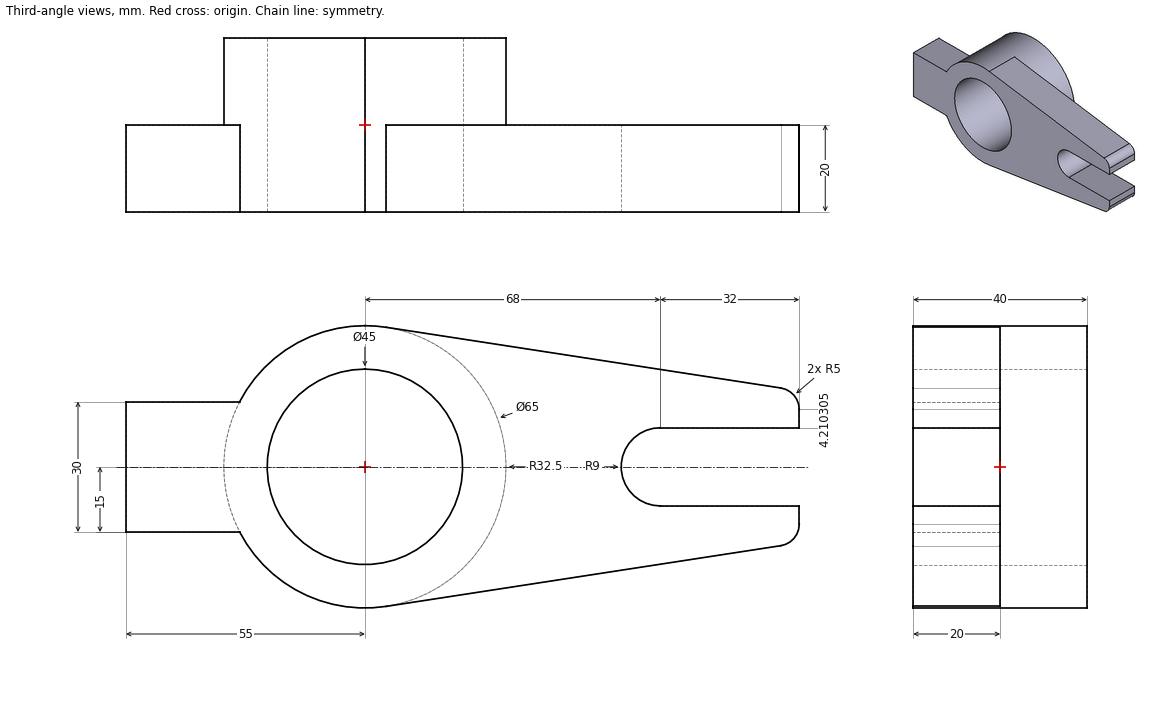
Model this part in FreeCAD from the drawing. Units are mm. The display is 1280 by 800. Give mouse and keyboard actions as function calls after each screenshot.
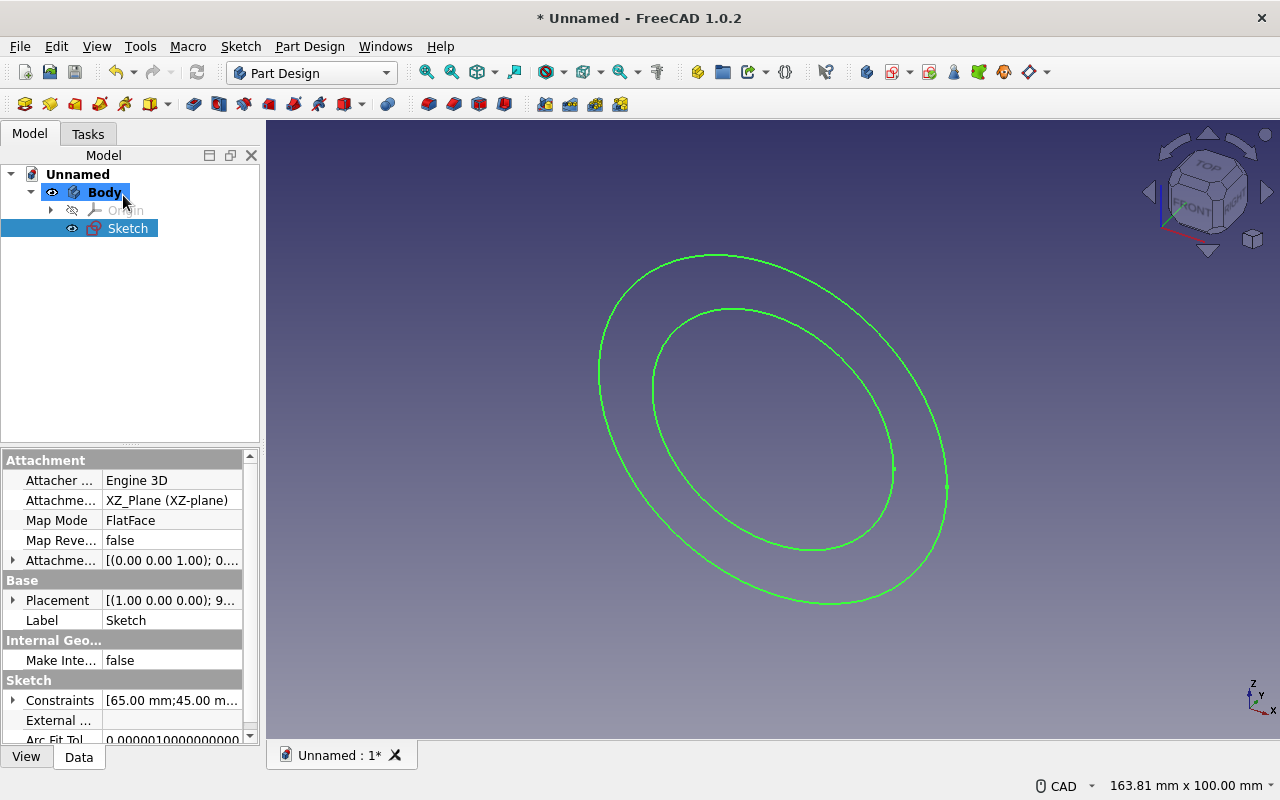
click(25, 104)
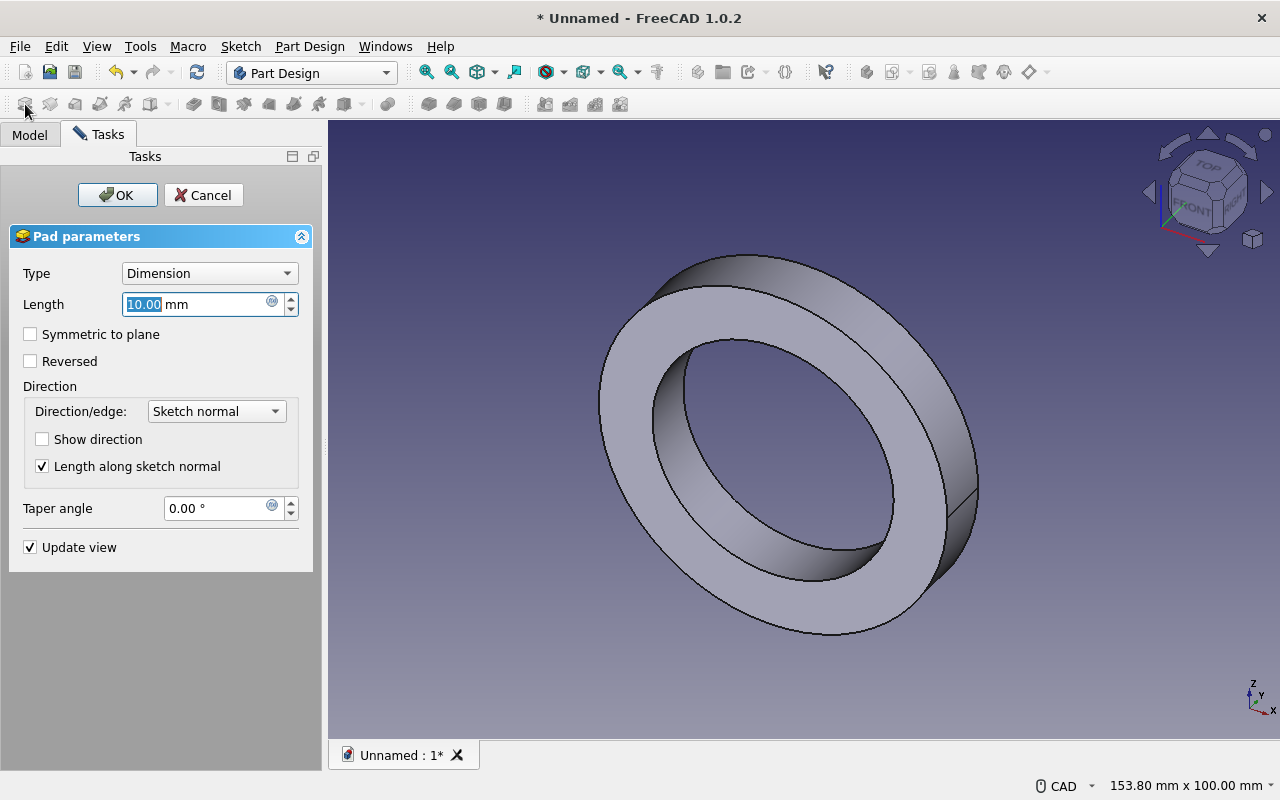
text(40)
key(Tab)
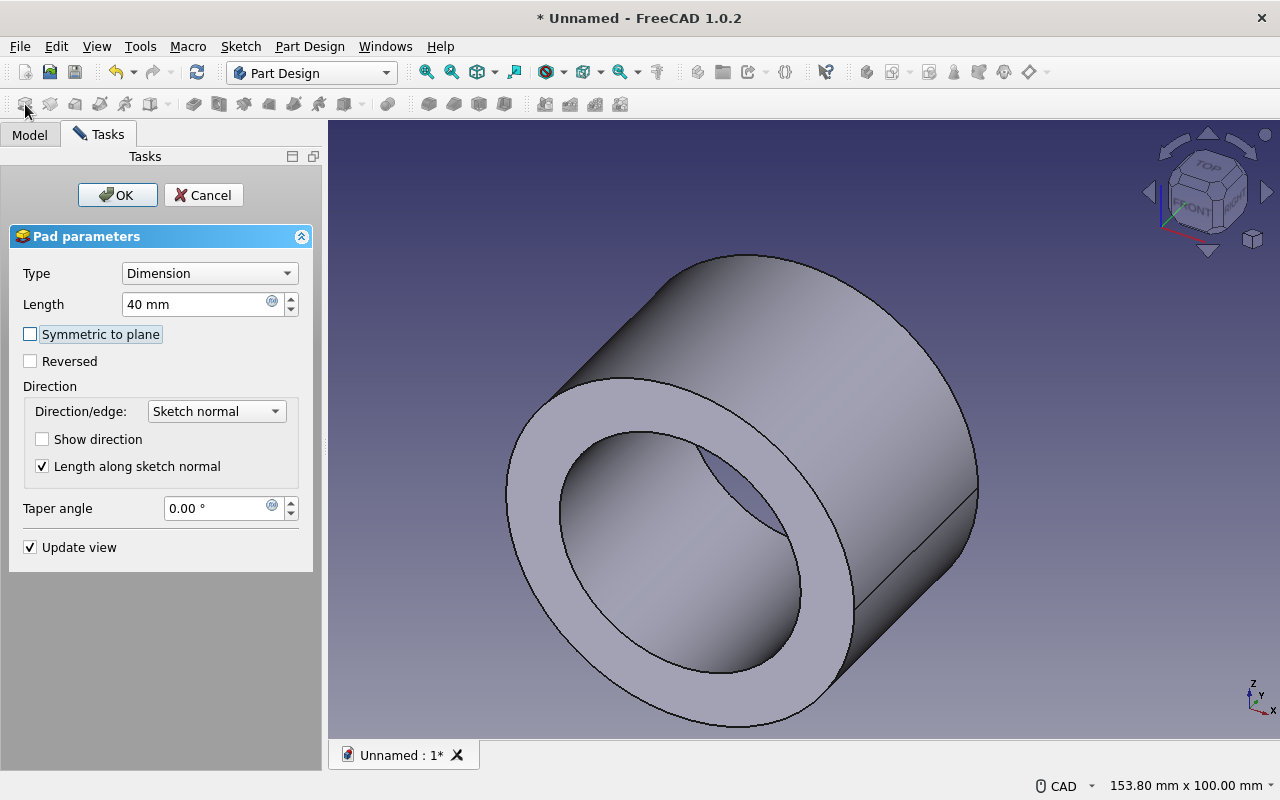
click(31, 334)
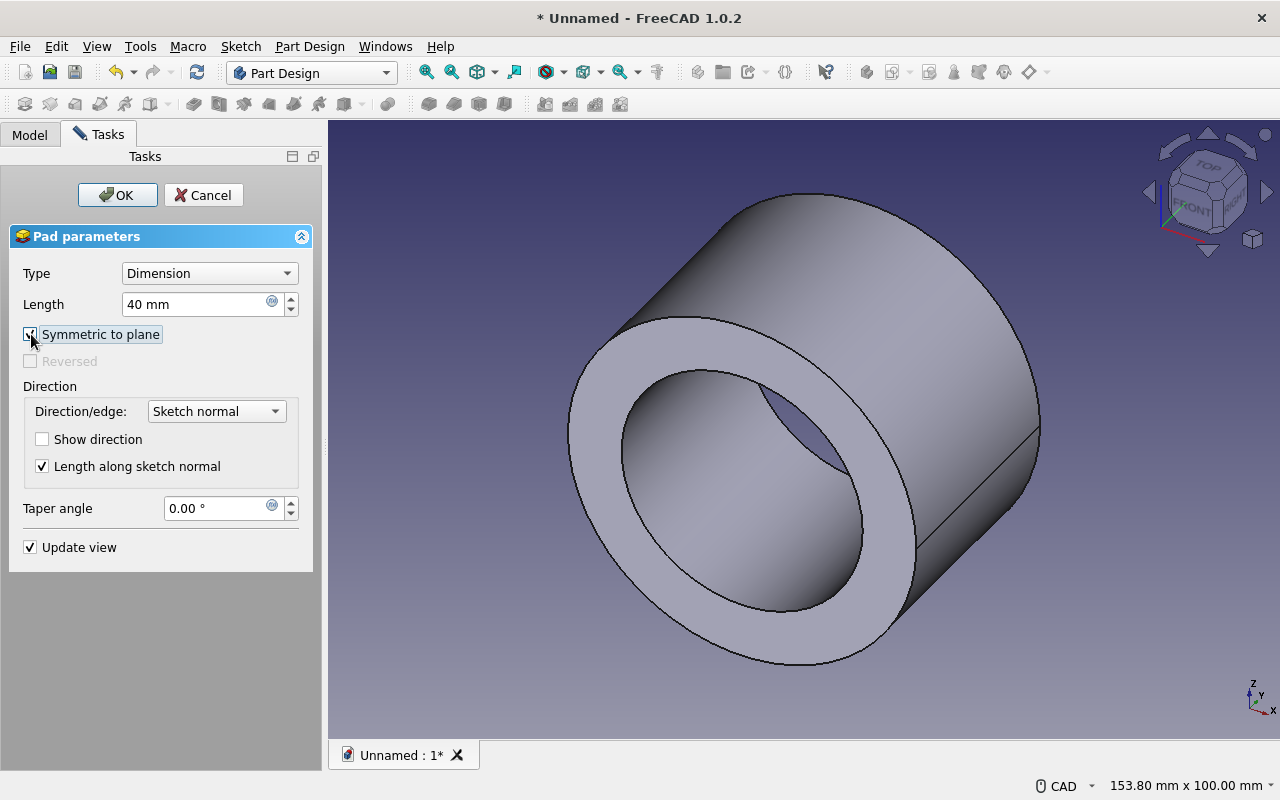
click(118, 195)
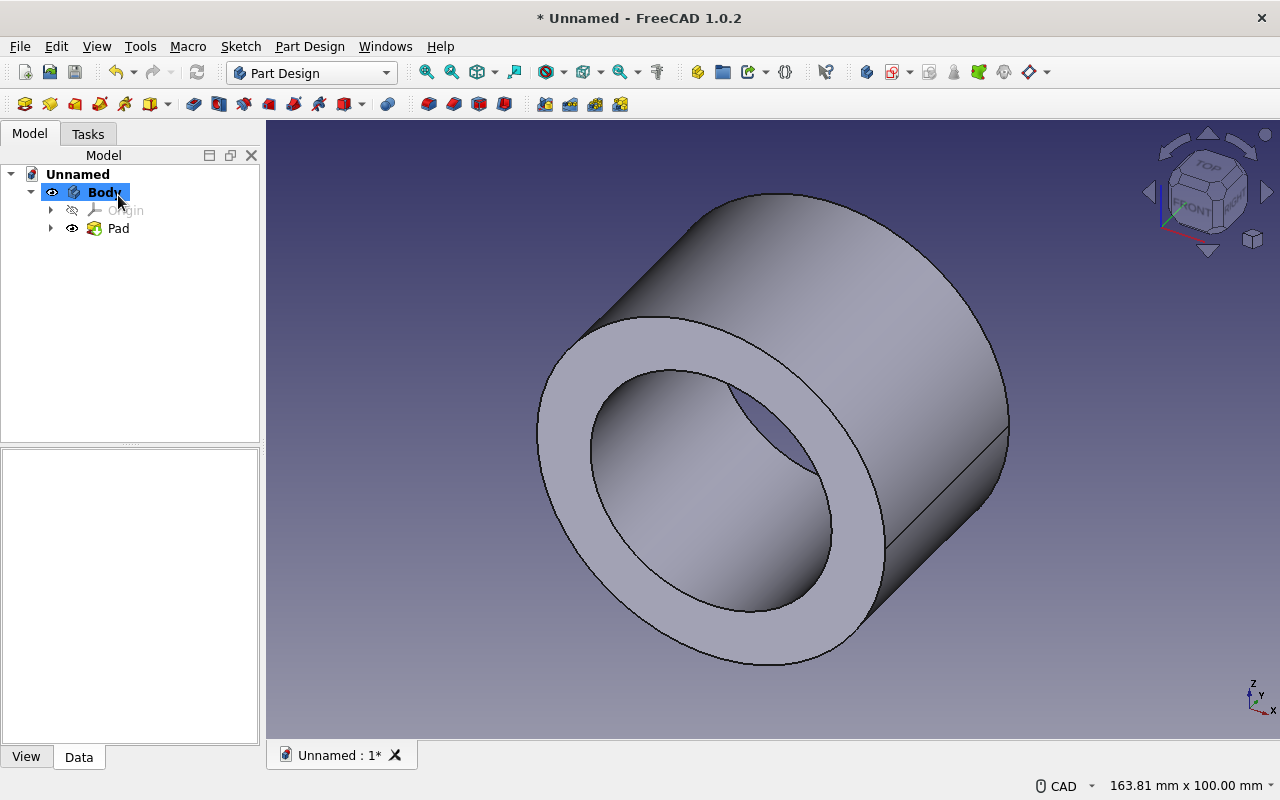
click(892, 72)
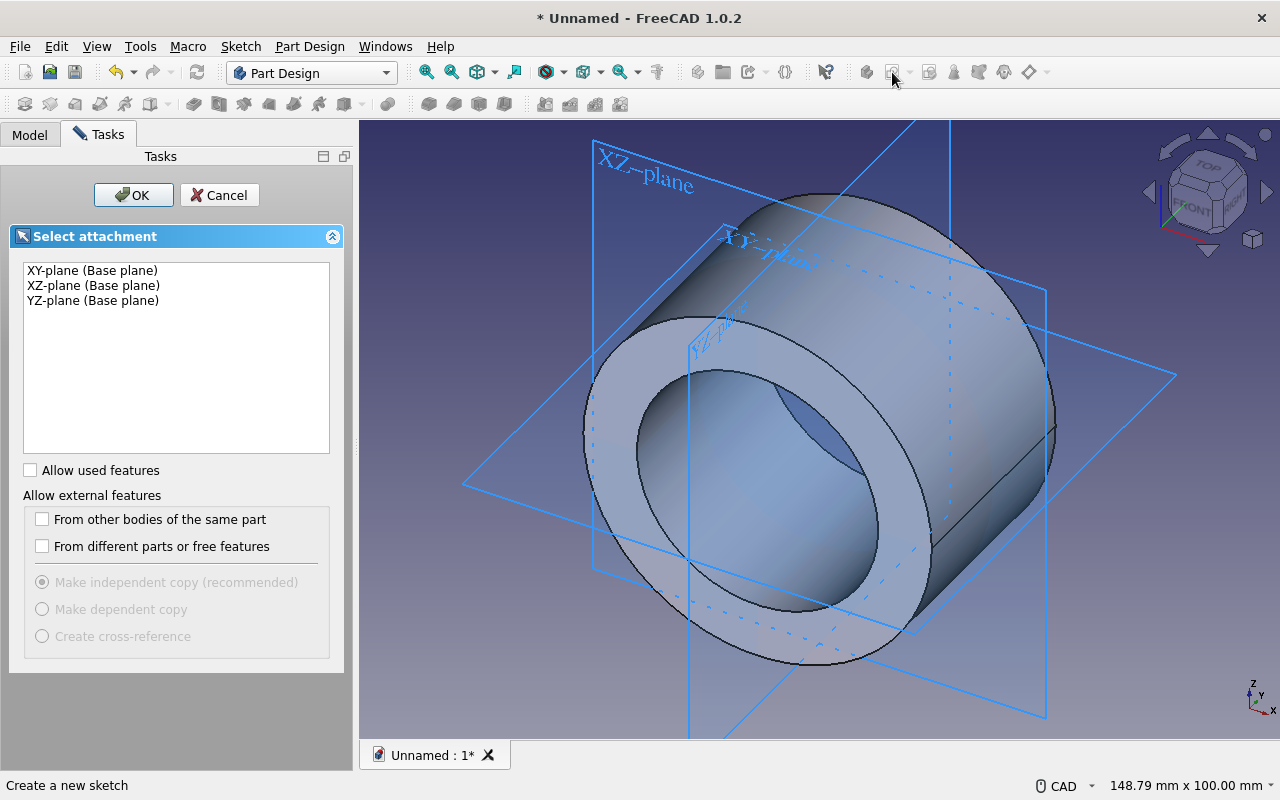
click(84, 286)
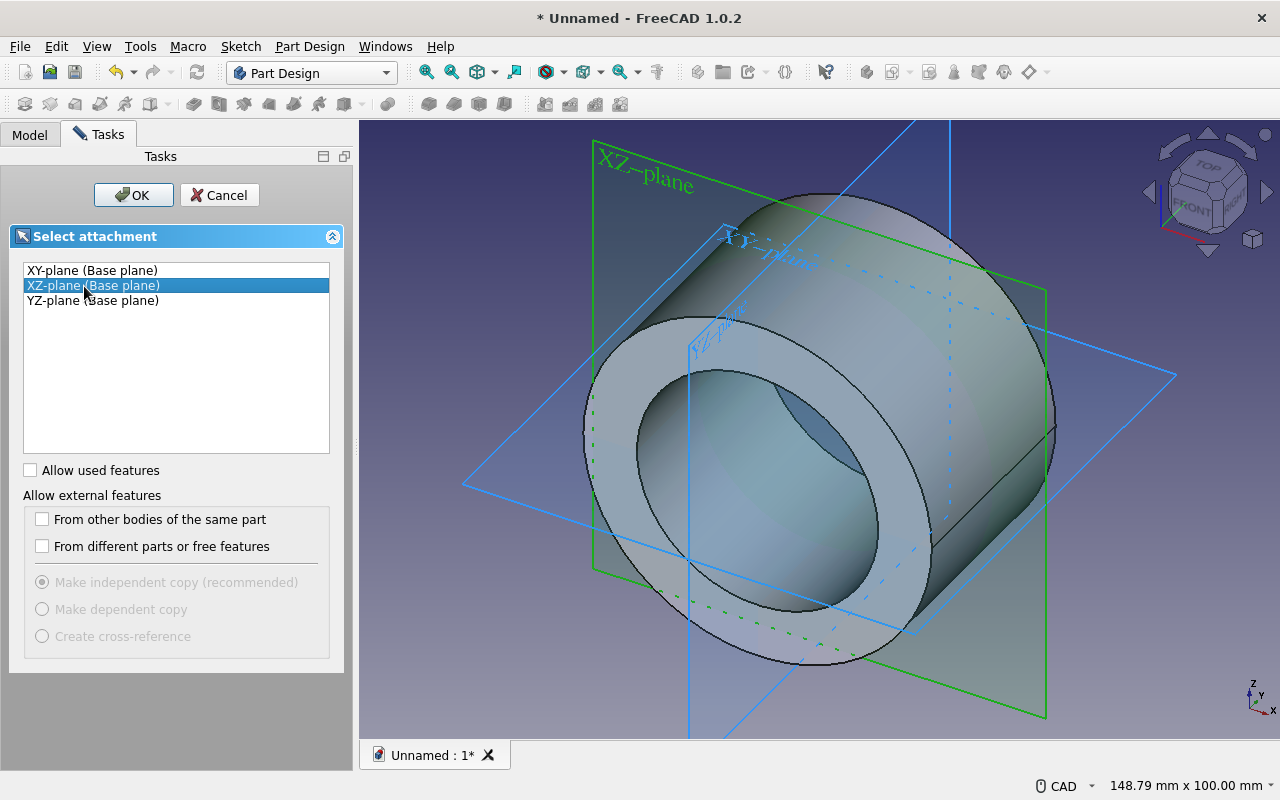
click(134, 195)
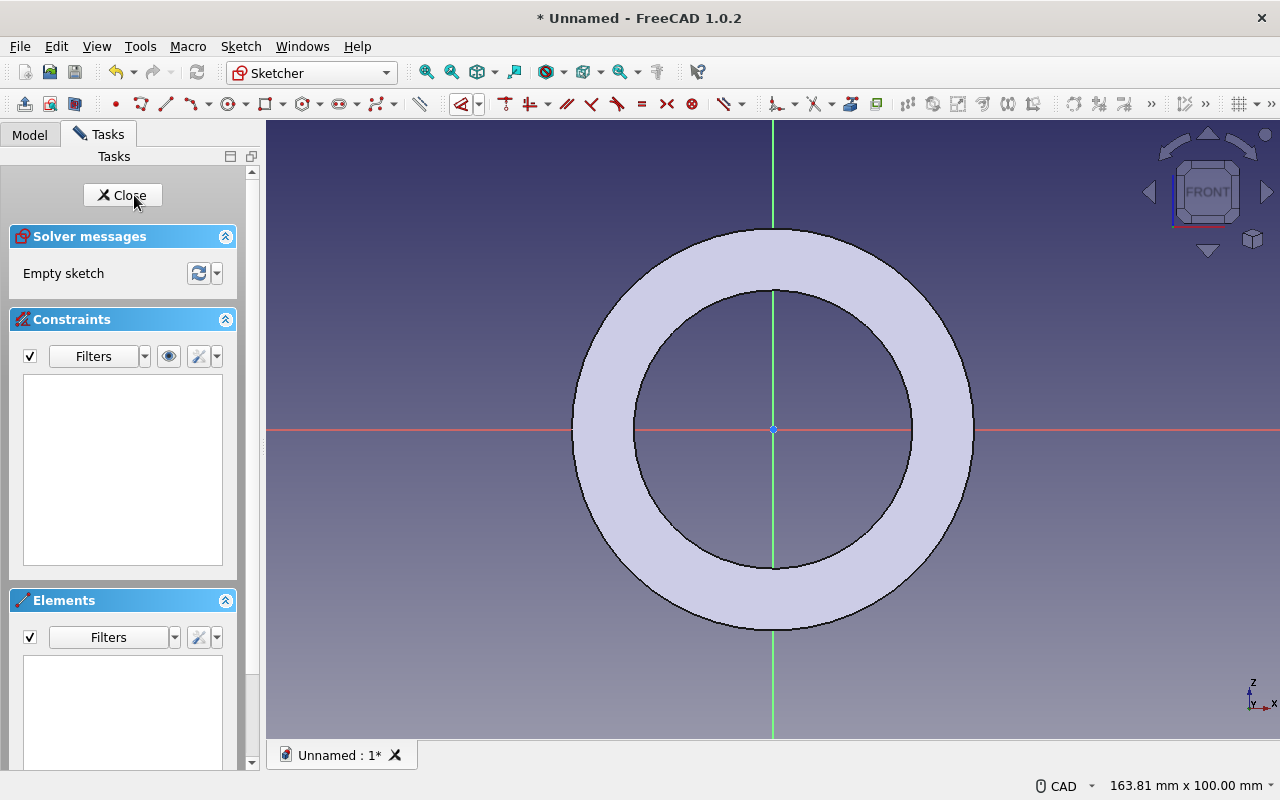
key(q)
key(s)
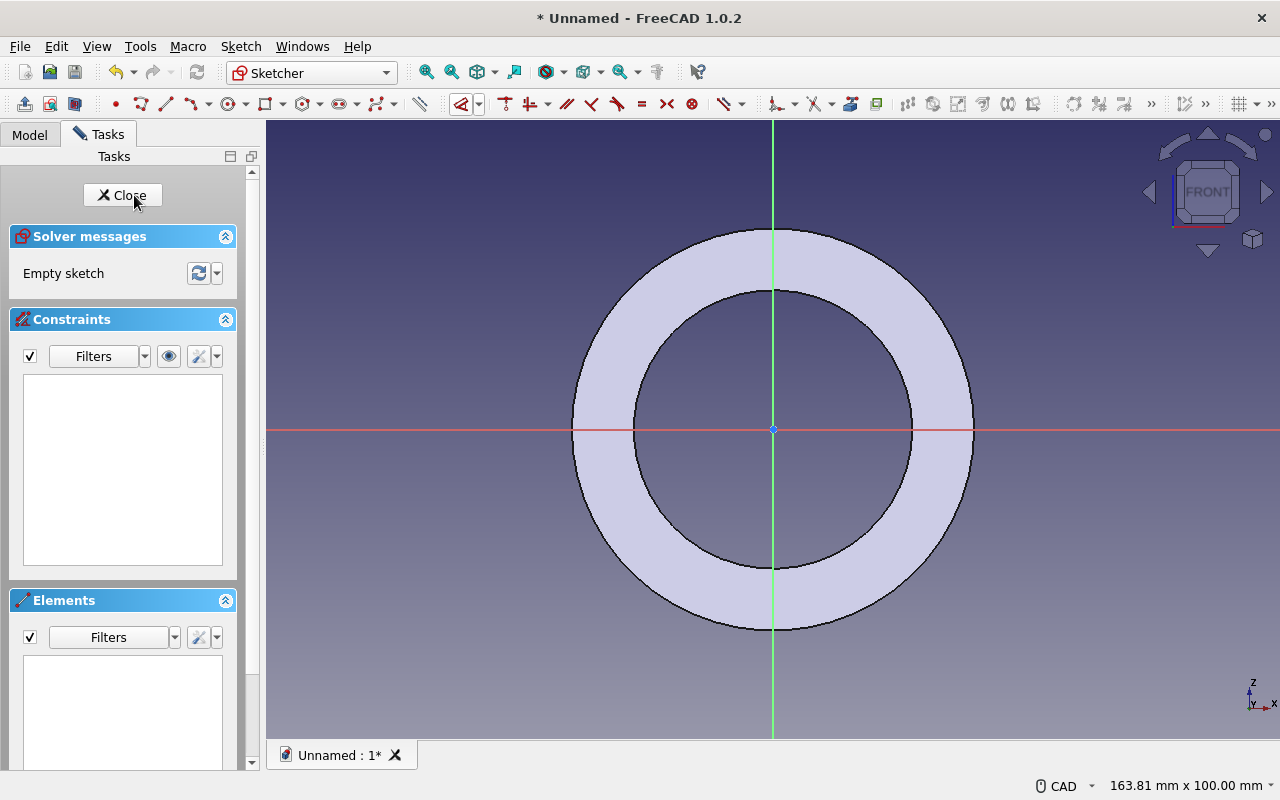
scroll(294, 429, down, 2)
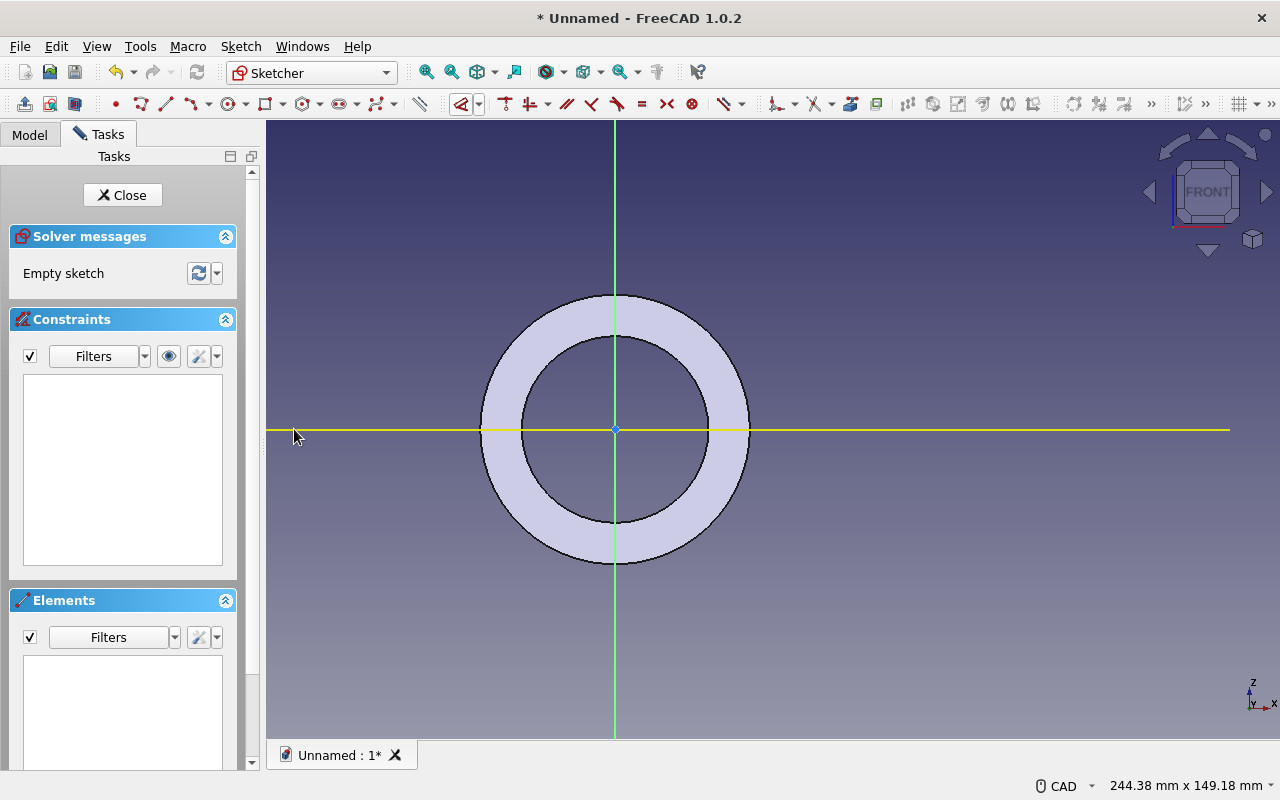
scroll(1063, 429, up, 2)